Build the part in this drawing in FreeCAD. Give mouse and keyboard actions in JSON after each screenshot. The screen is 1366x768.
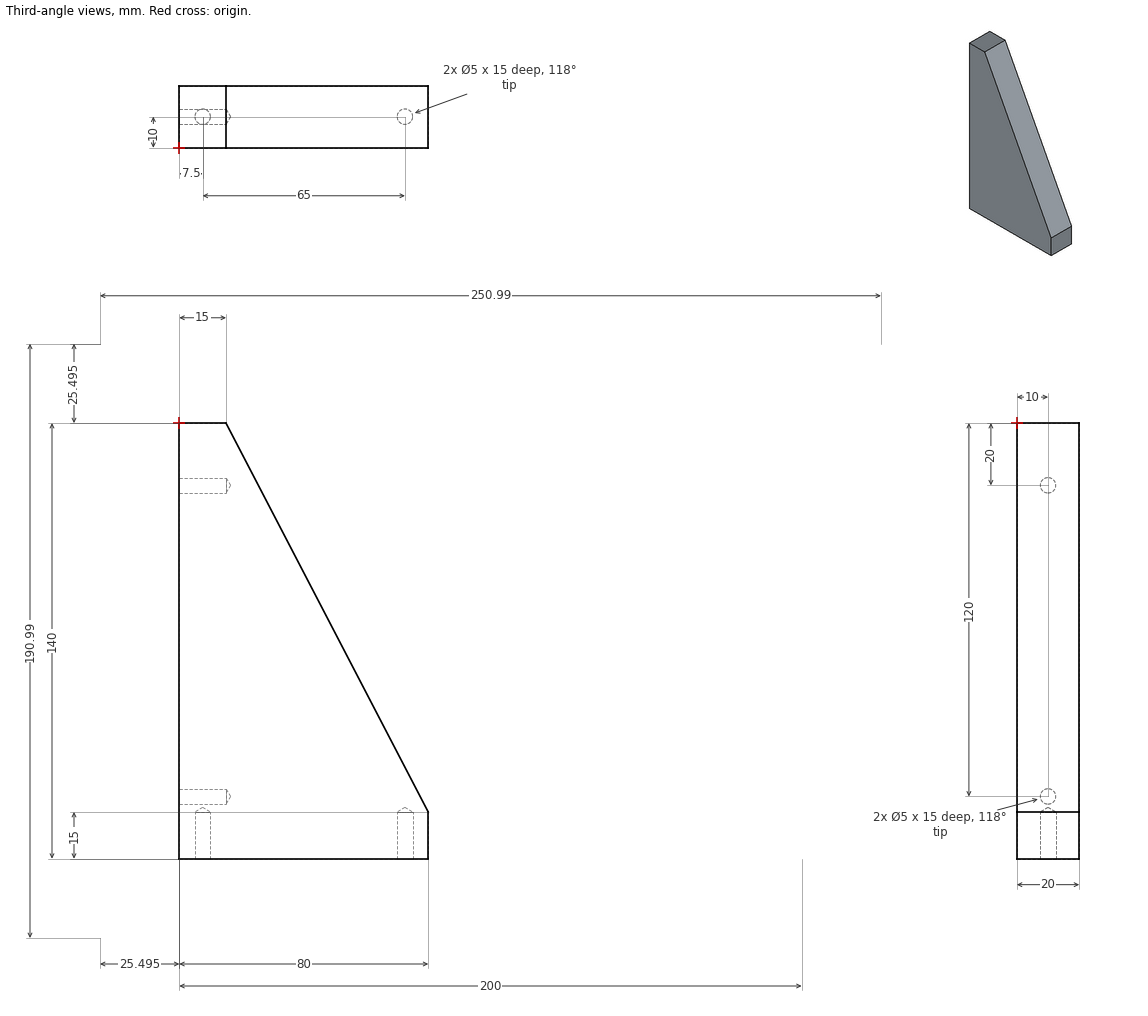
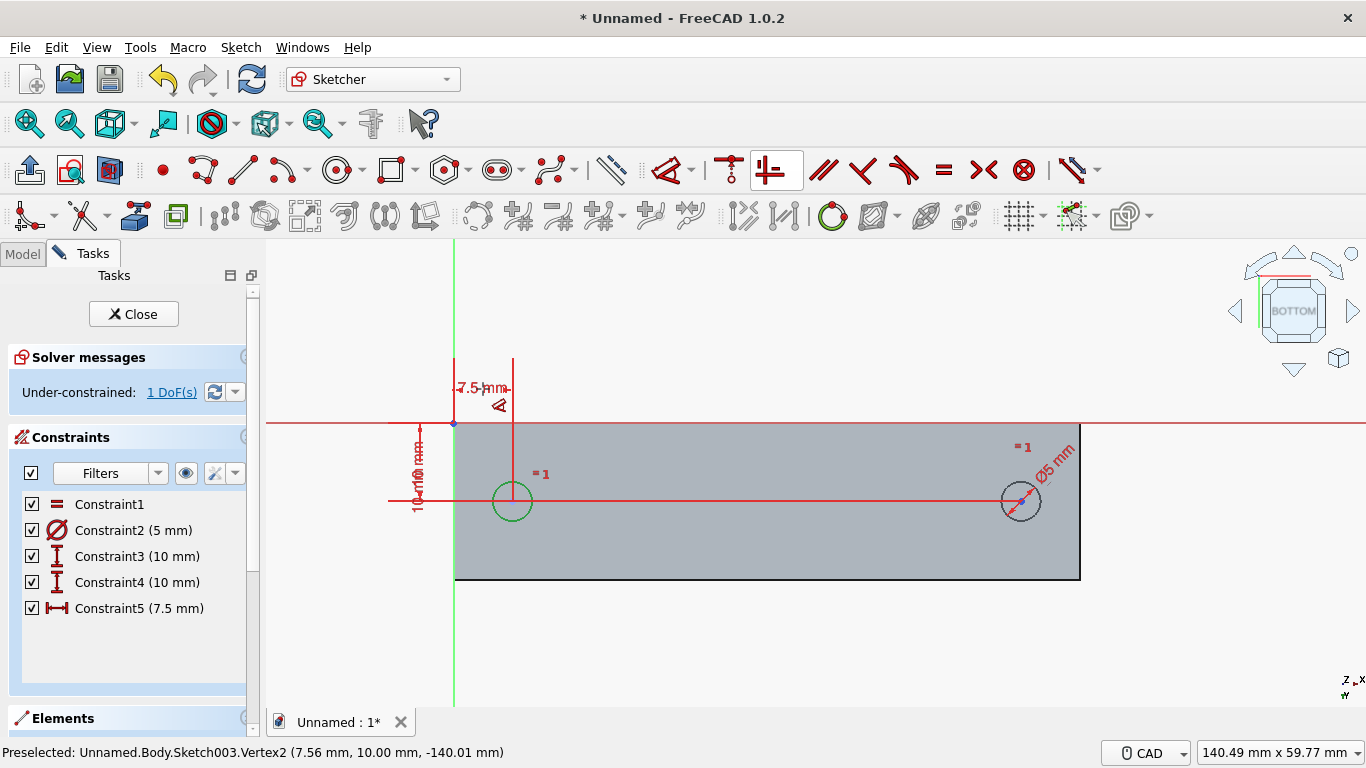
{"action": "left_click", "coordinate": [1021, 501]}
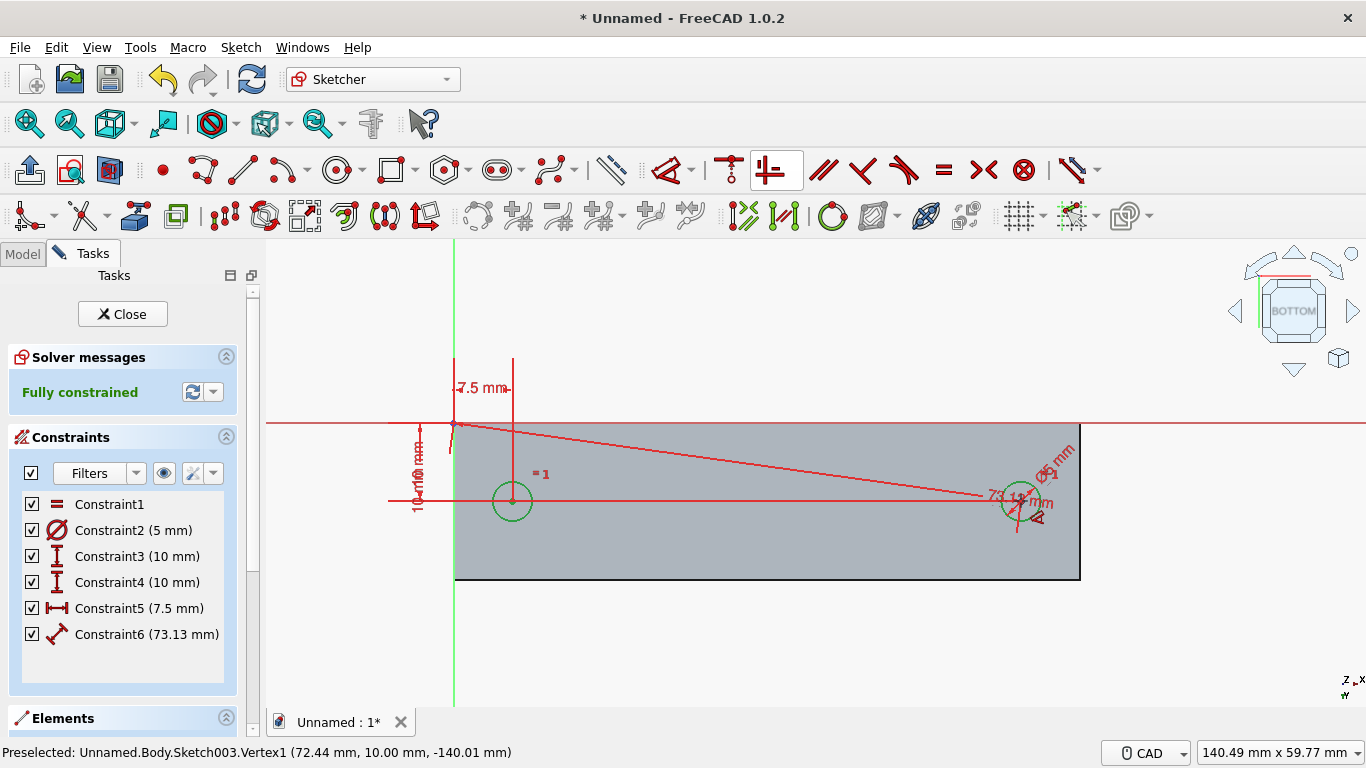
{"action": "left_click", "coordinate": [513, 501]}
{"action": "left_click", "coordinate": [767, 535]}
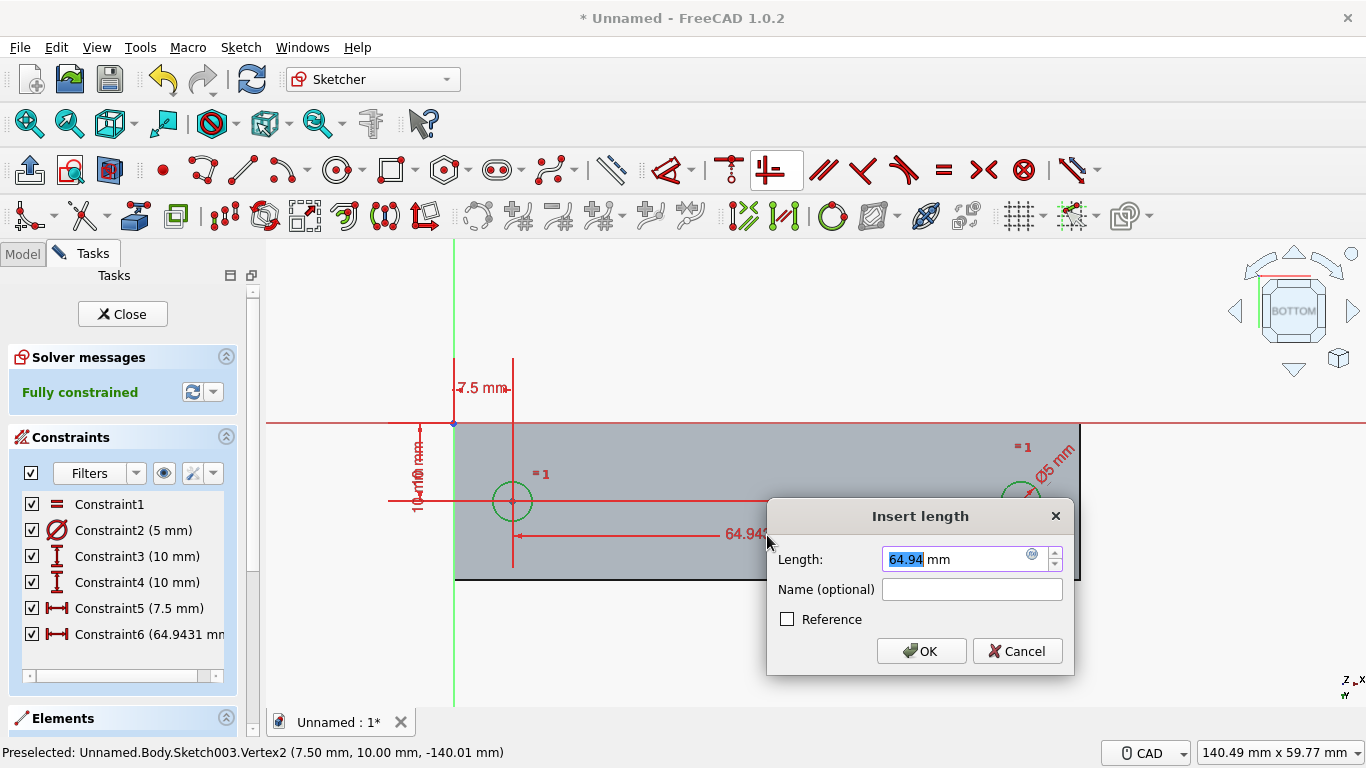
{"action": "type", "text": "65"}
{"action": "key", "text": "Return"}
{"action": "key", "text": "Escape"}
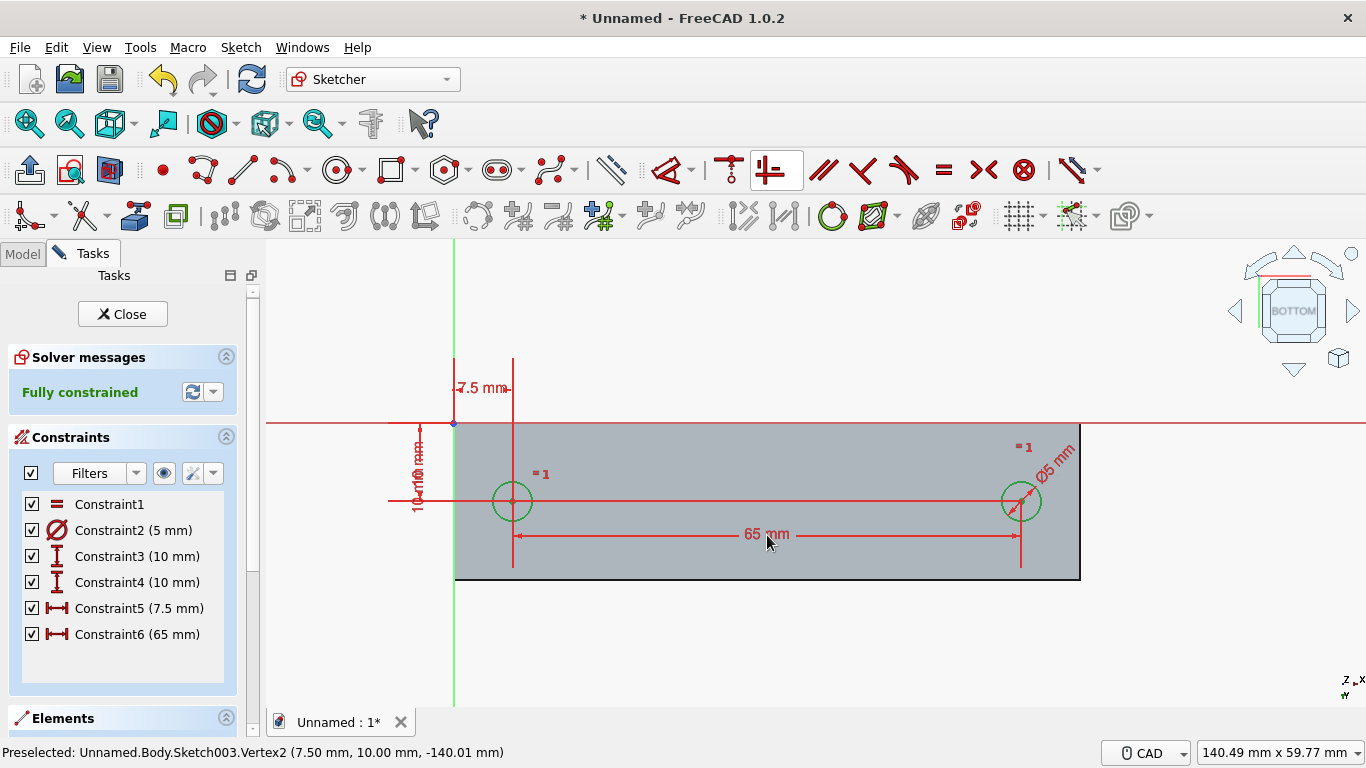
{"action": "left_click", "coordinate": [123, 314]}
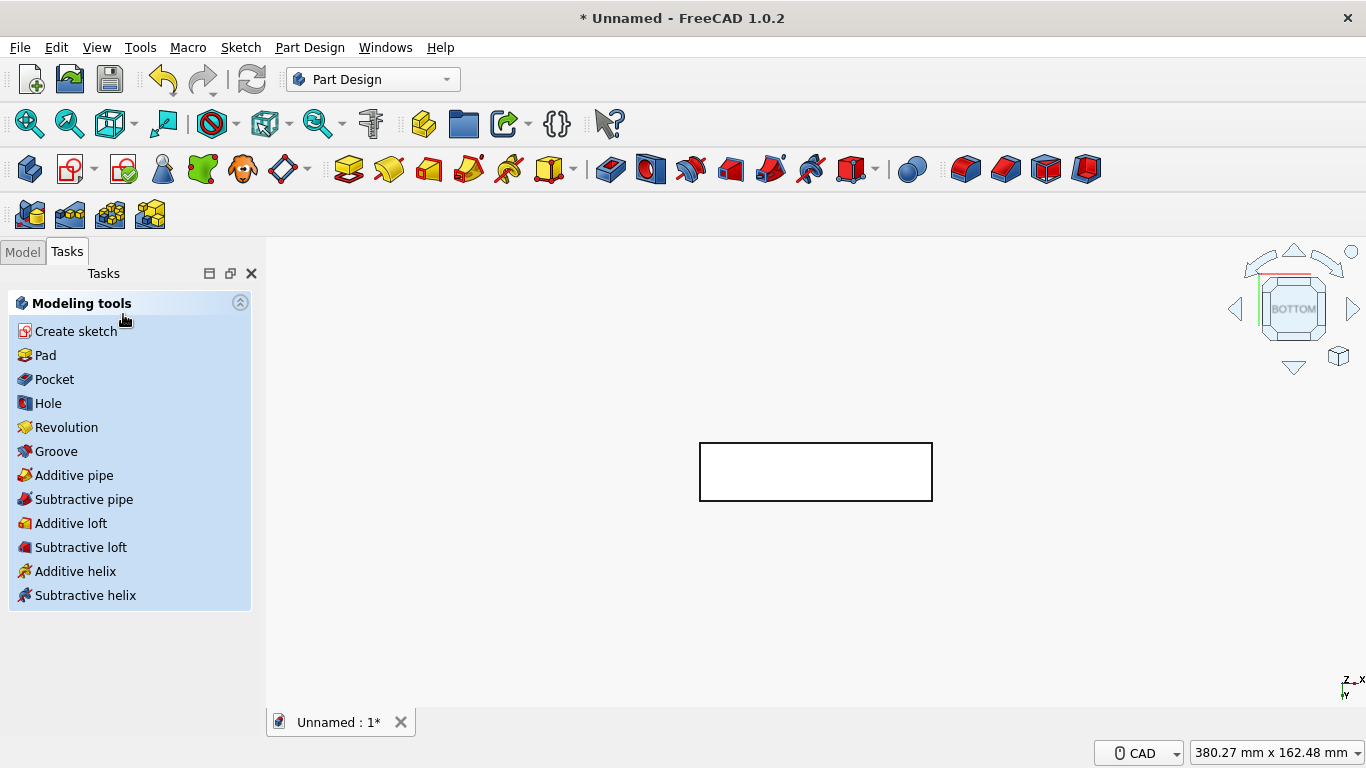
{"action": "left_click", "coordinate": [652, 170]}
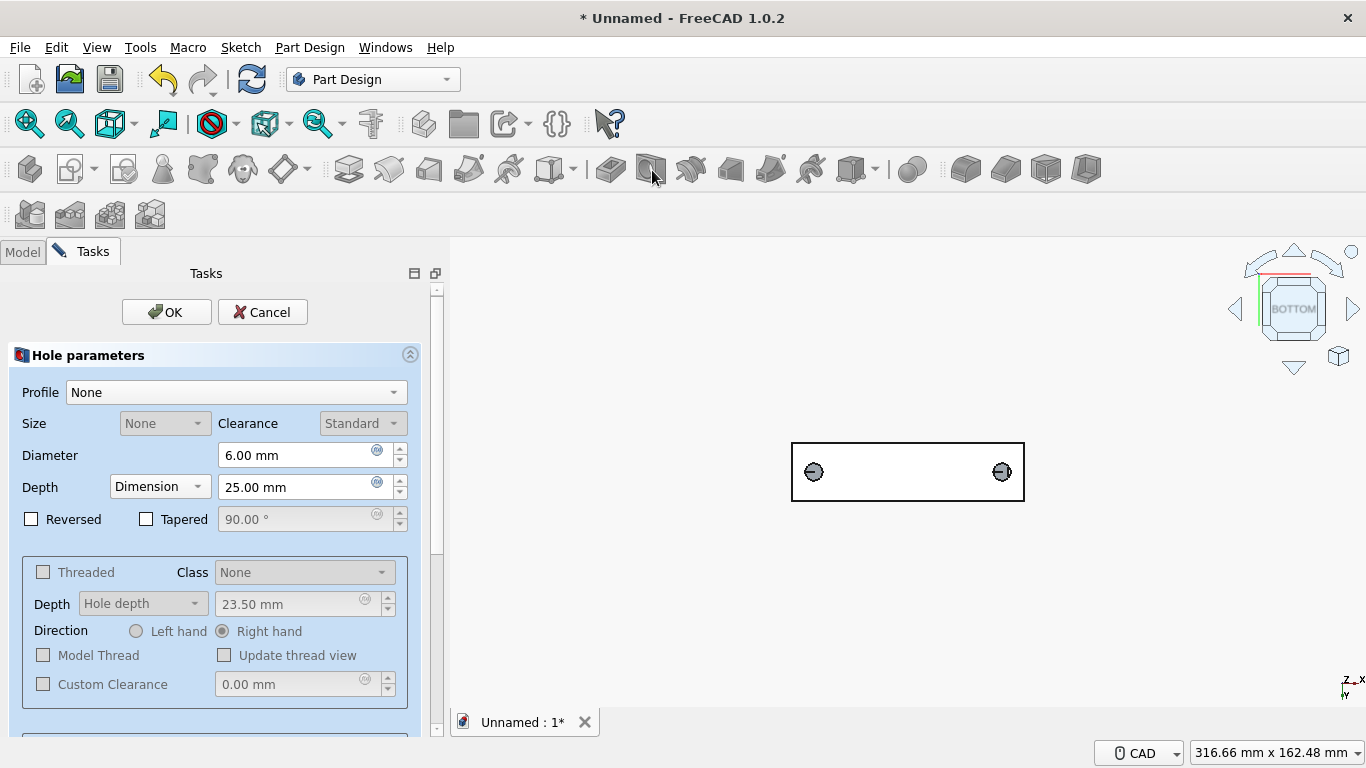
{"action": "triple_click", "coordinate": [305, 455]}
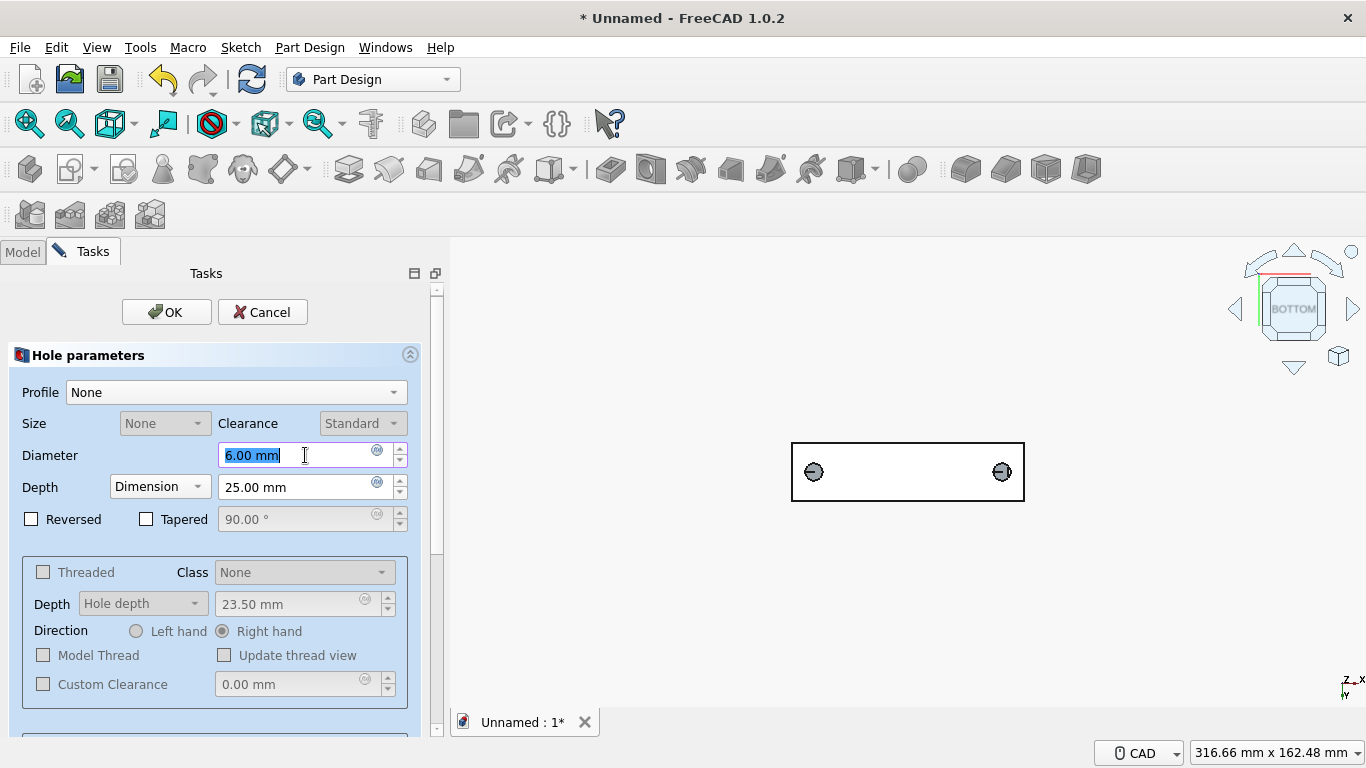
{"action": "type", "text": "5"}
{"action": "key", "text": "Tab"}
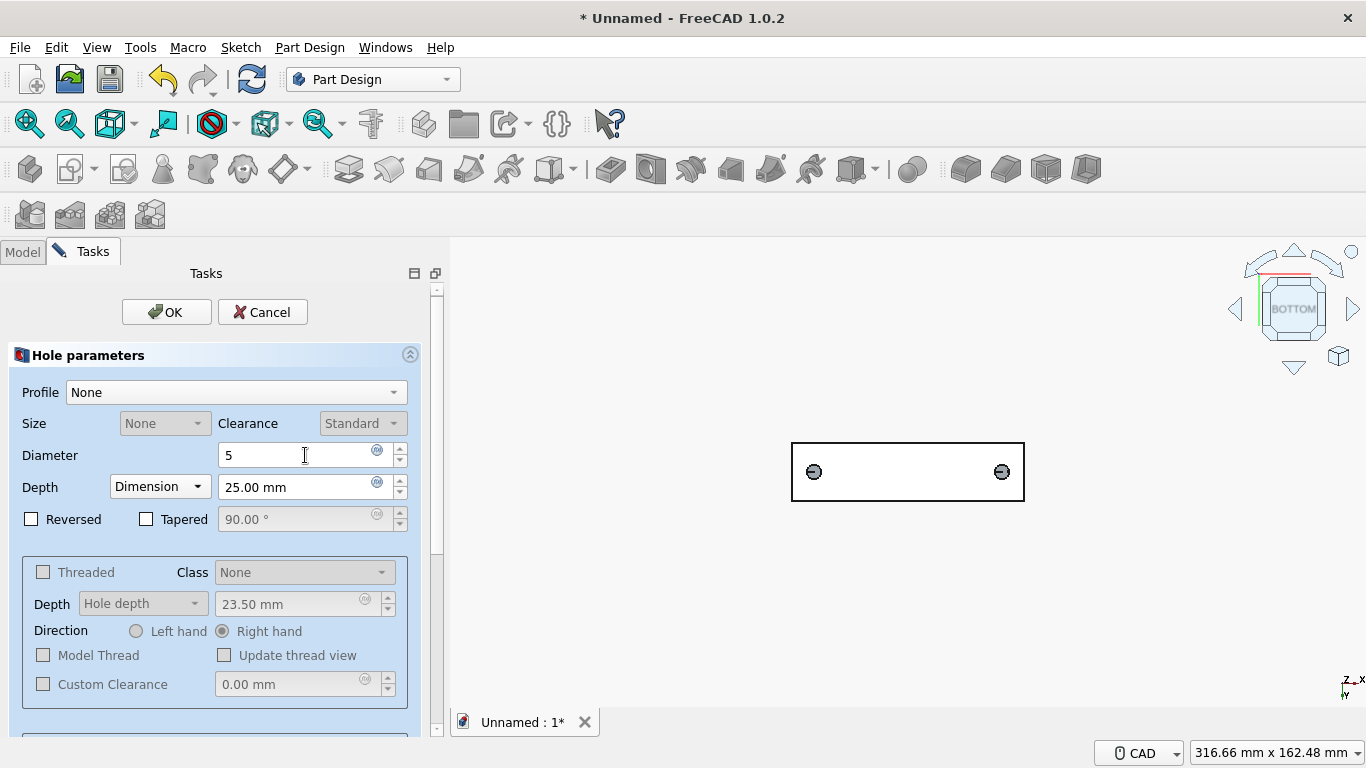
{"action": "triple_click", "coordinate": [305, 487]}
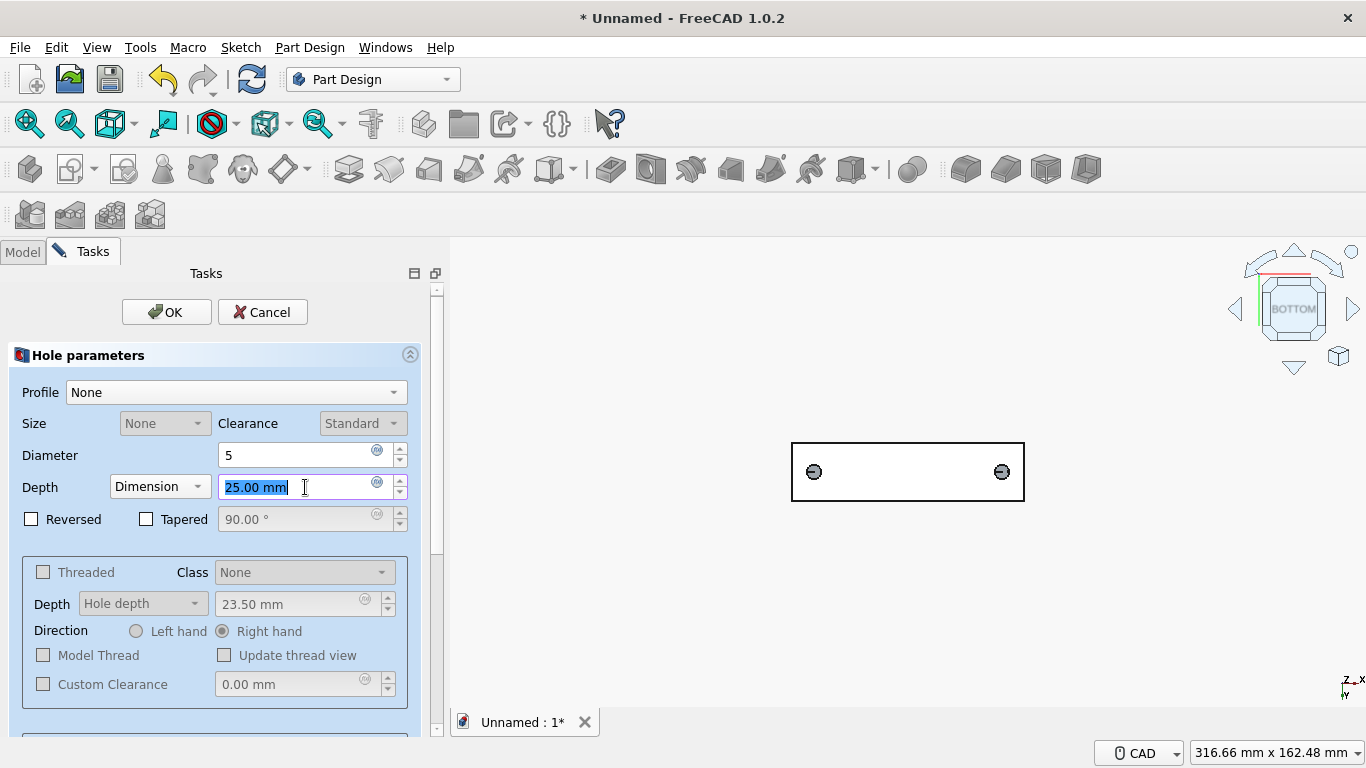
{"action": "type", "text": "15"}
{"action": "key", "text": "Tab"}